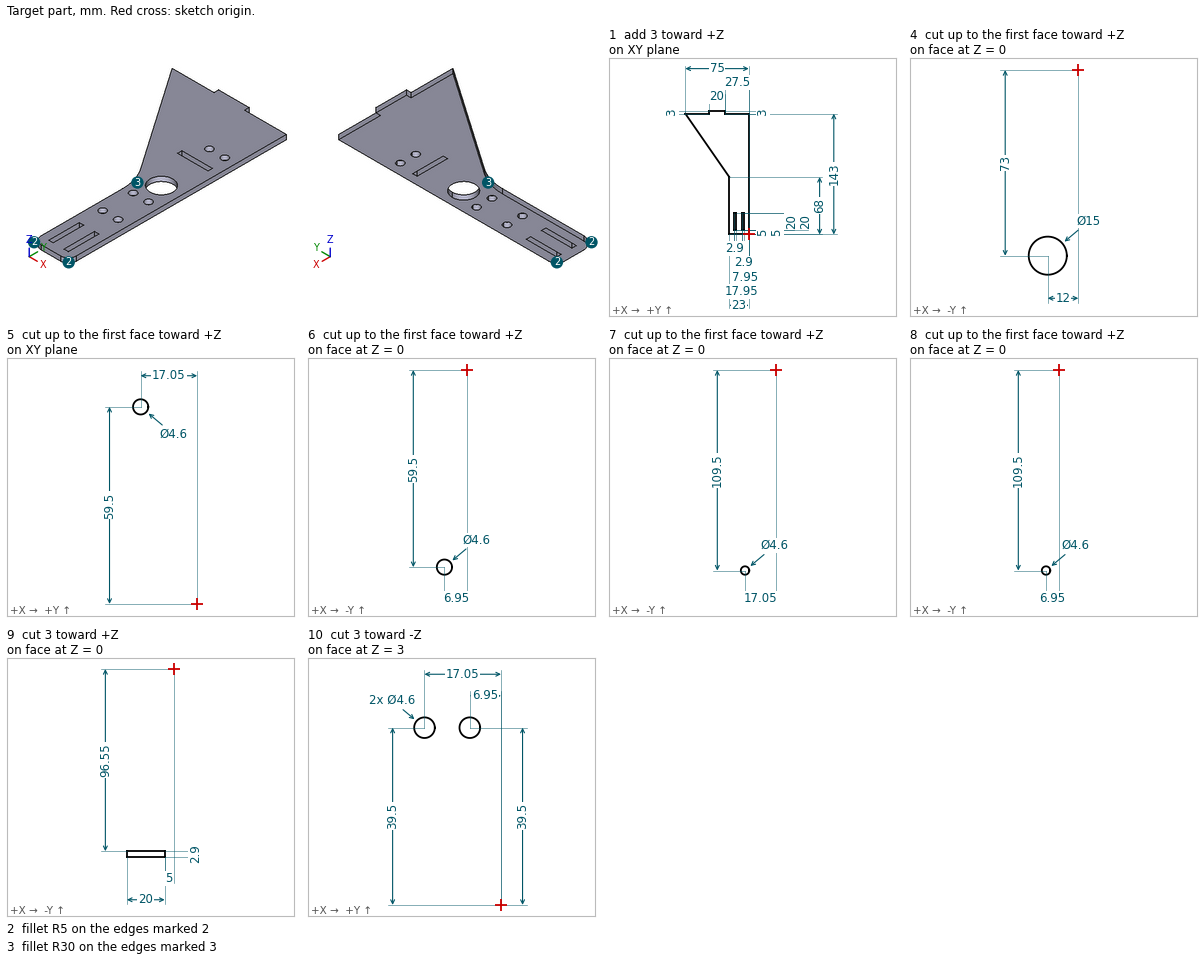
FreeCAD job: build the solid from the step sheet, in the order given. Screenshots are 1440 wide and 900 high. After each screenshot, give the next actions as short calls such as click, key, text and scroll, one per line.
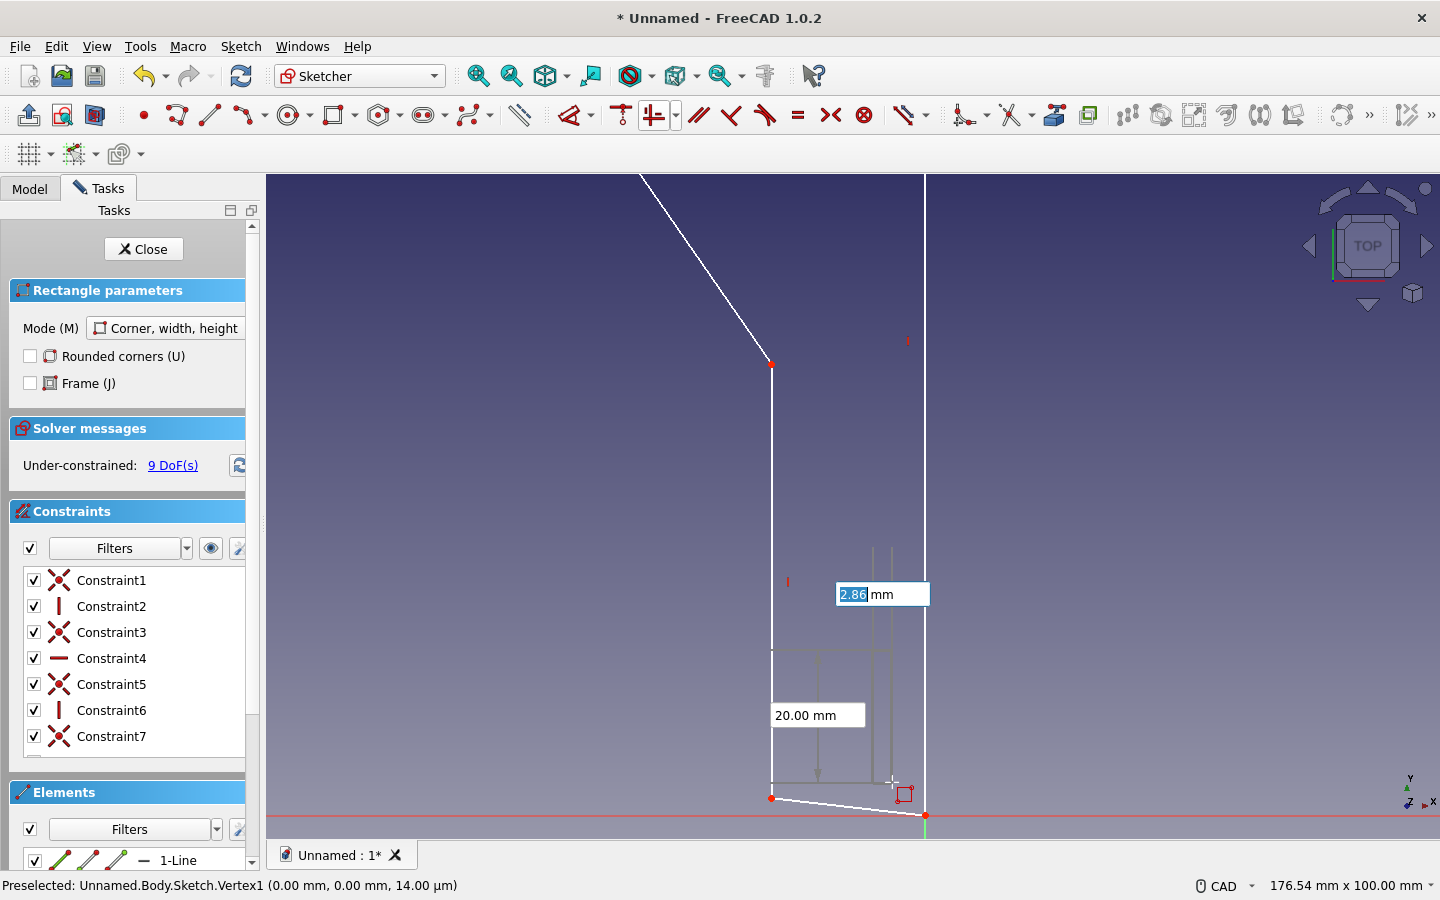
text(2.9)
key(Tab)
text(20)
key(Return)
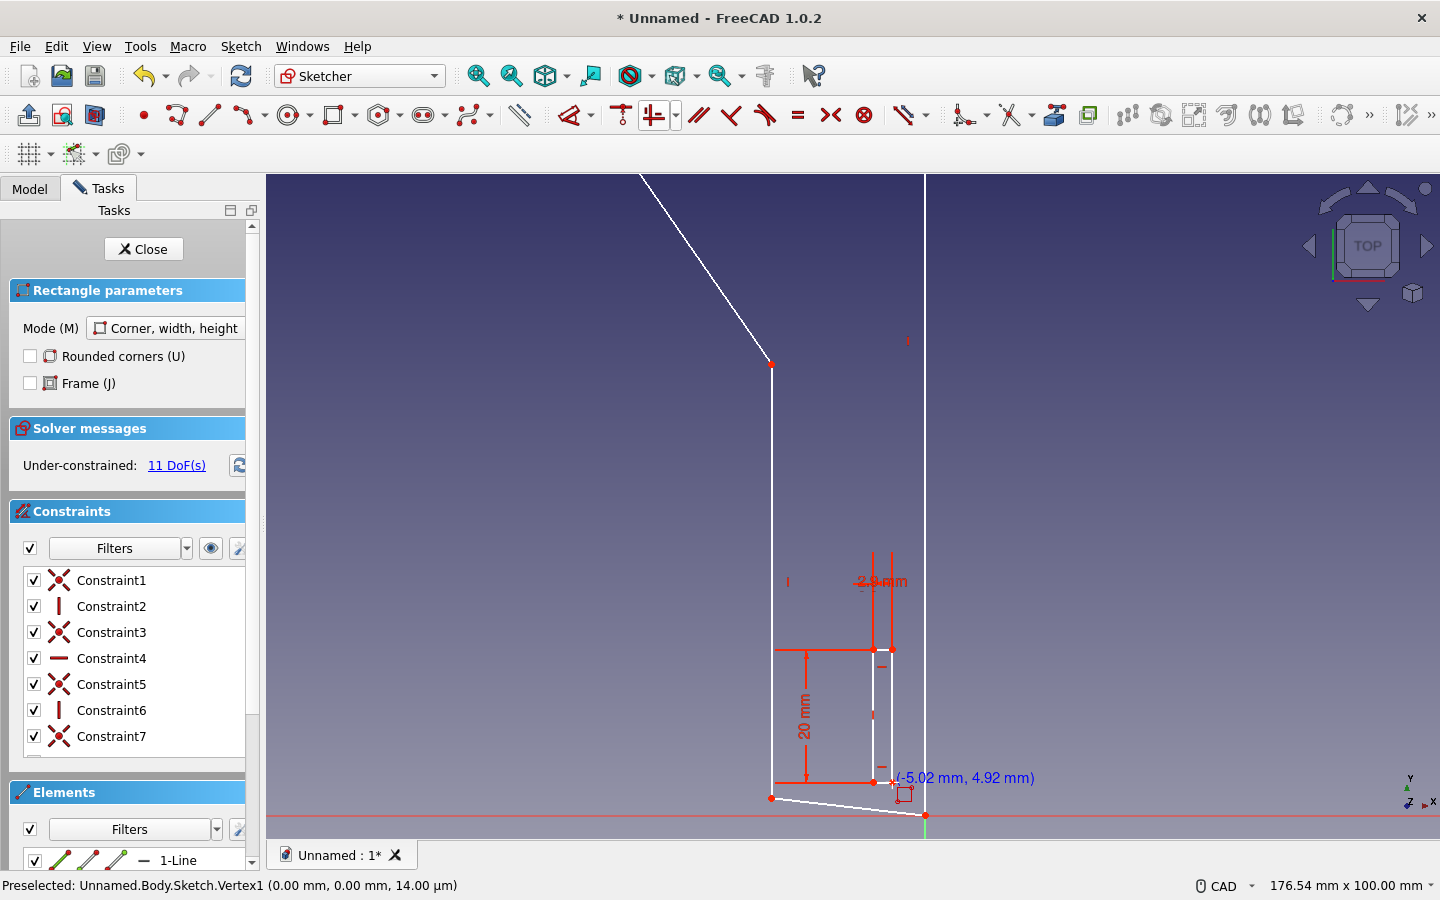
click(806, 649)
move(825, 782)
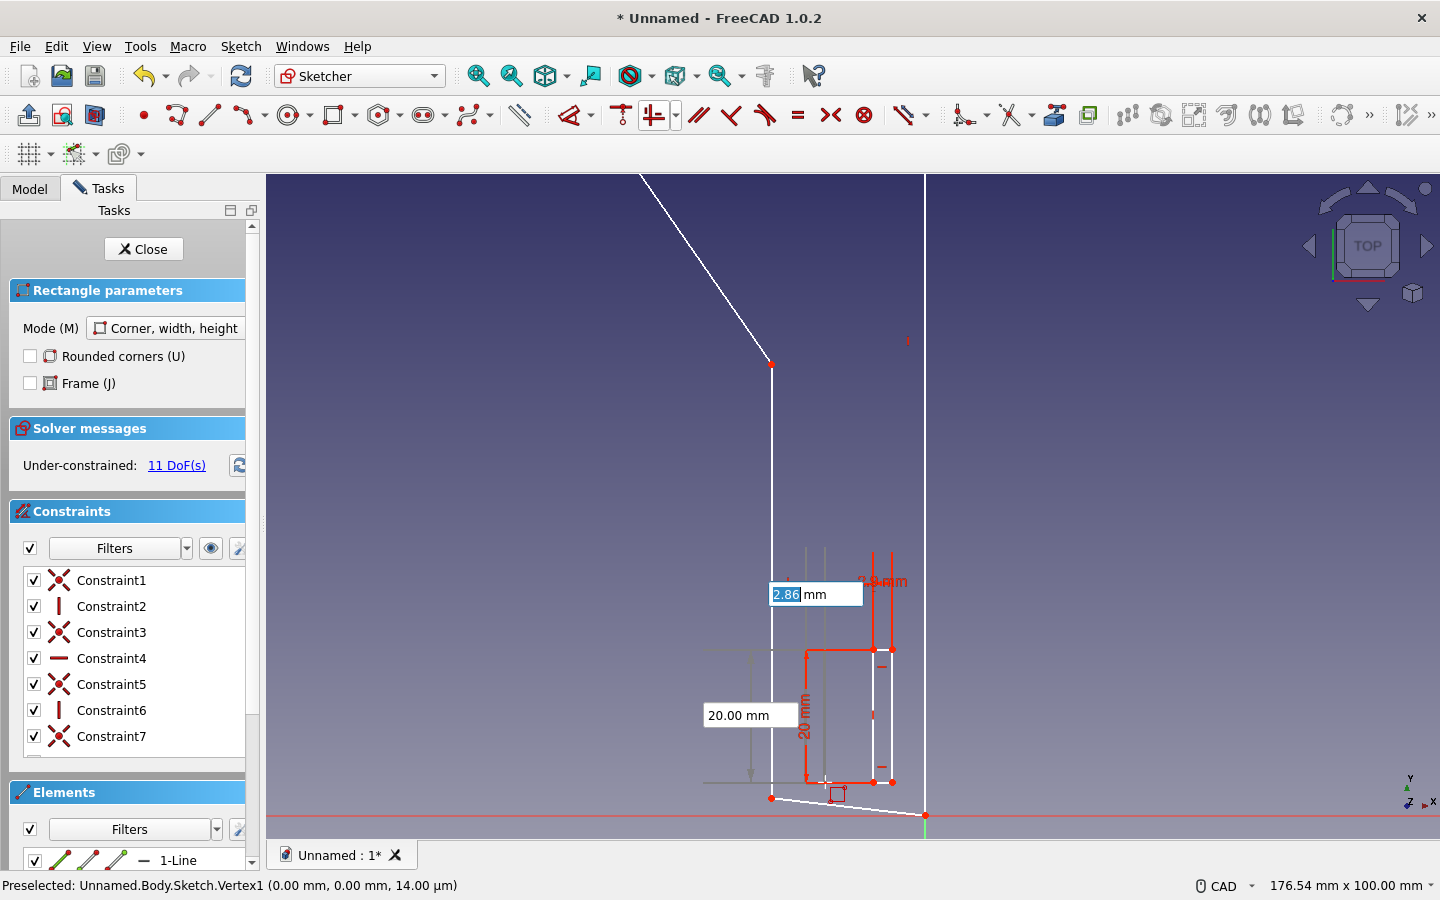
text(2.9)
key(Tab)
text(20)
key(Return)
key(Escape)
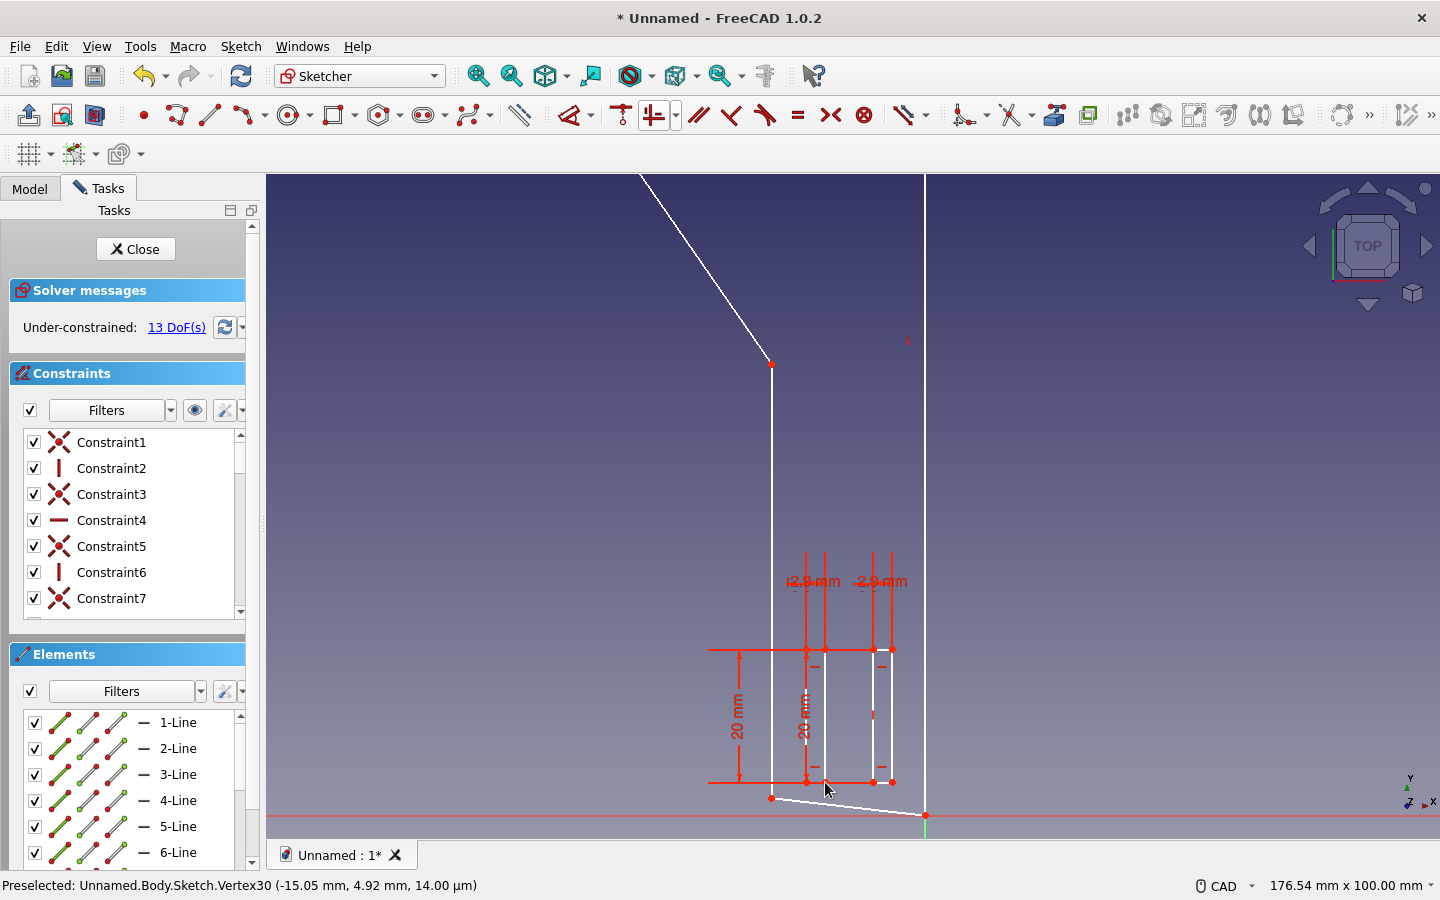
click(818, 803)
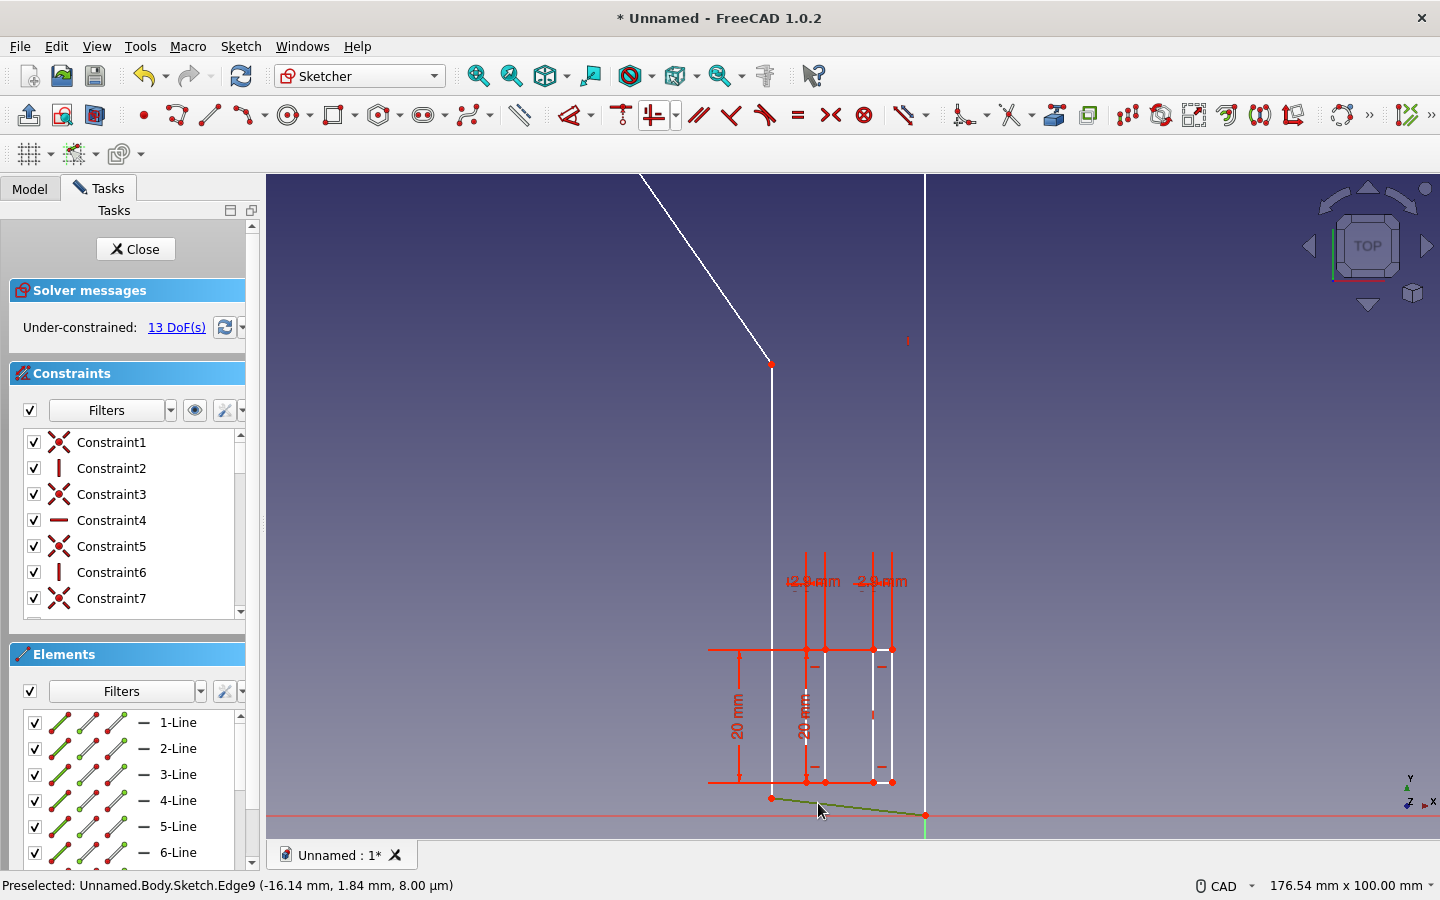
key(h)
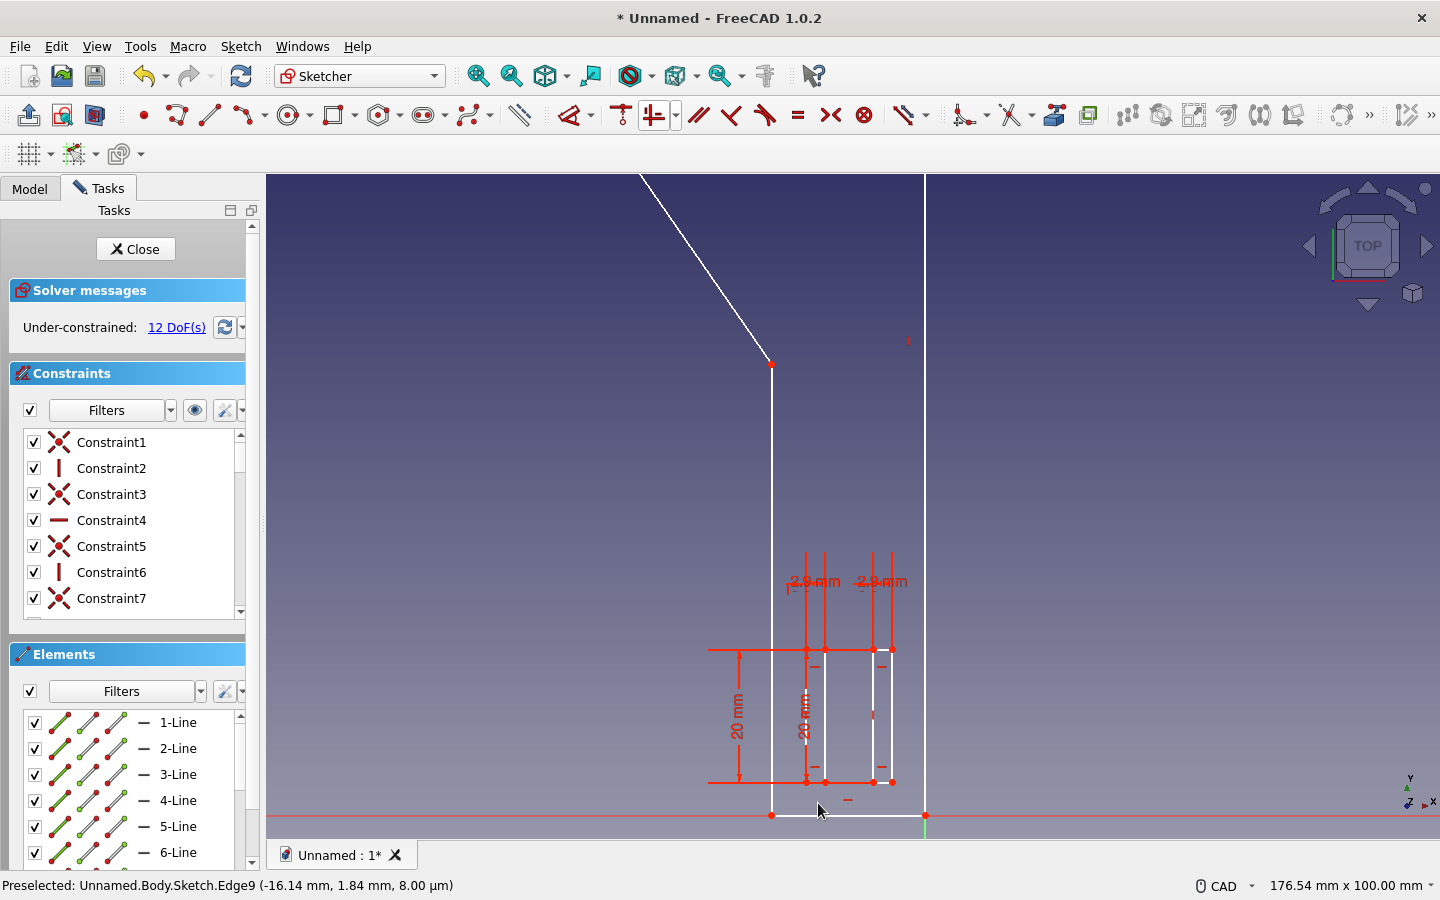
key(d)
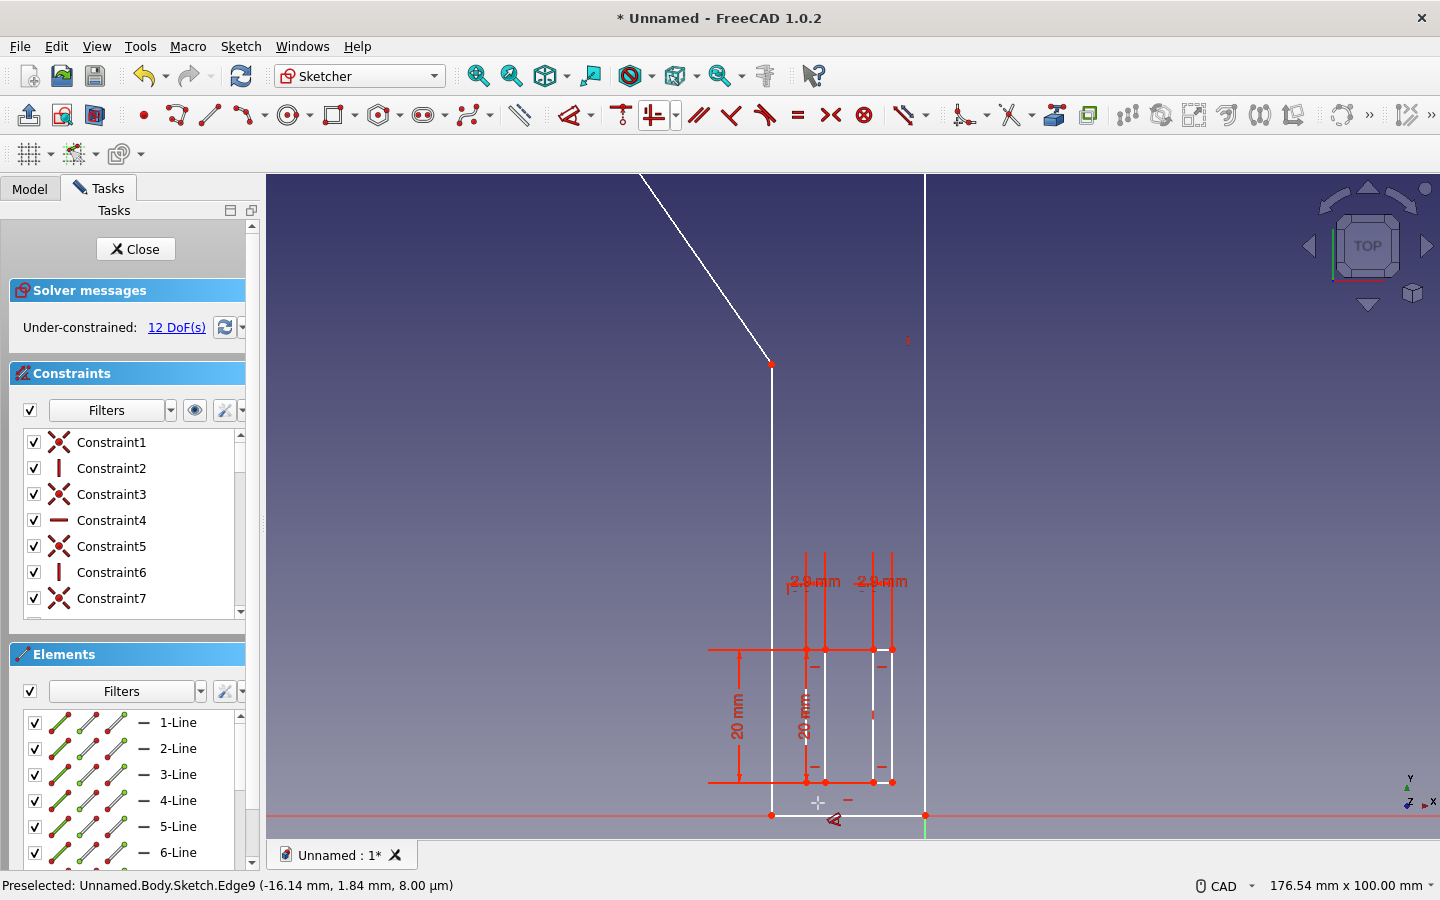
scroll(873, 650, down, 4)